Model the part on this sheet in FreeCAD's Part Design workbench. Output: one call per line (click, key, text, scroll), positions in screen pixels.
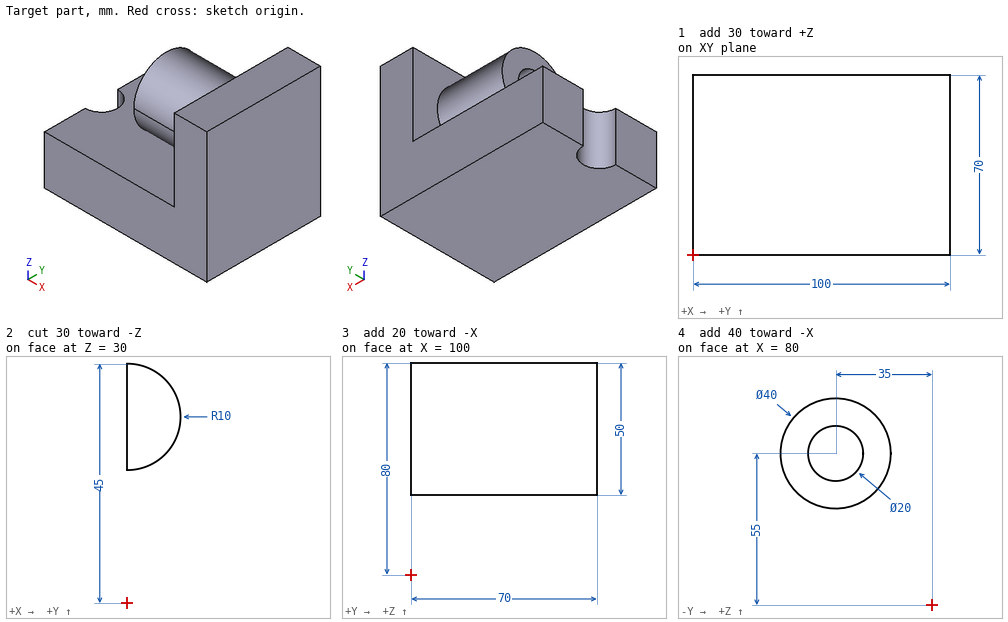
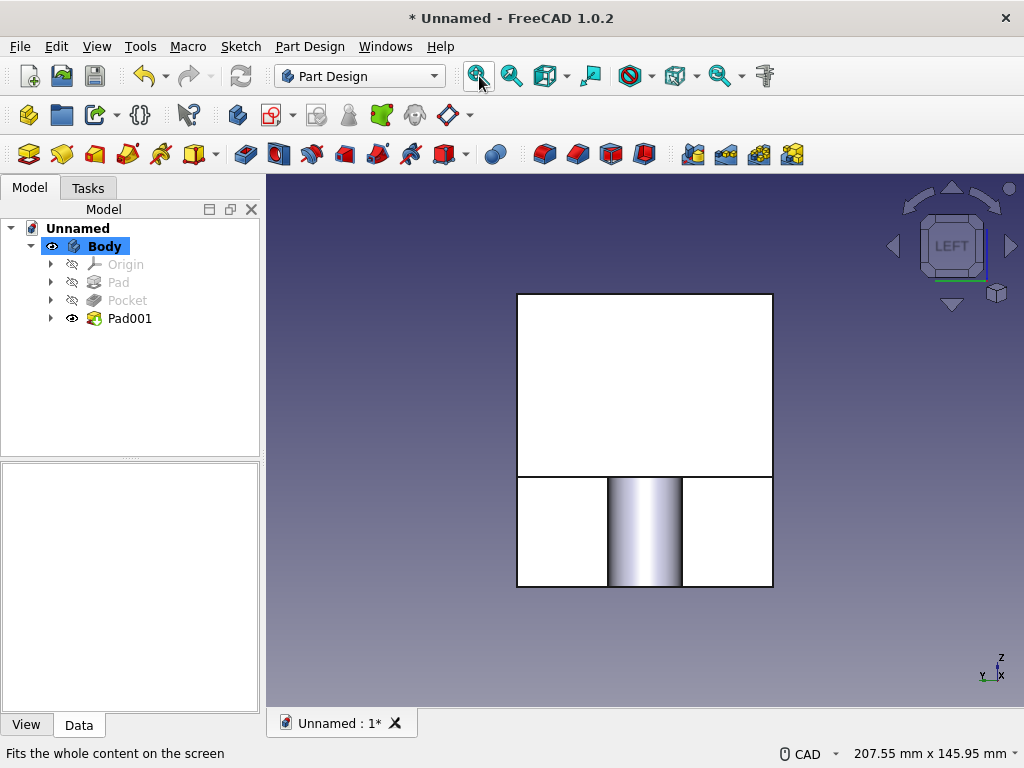
click(608, 385)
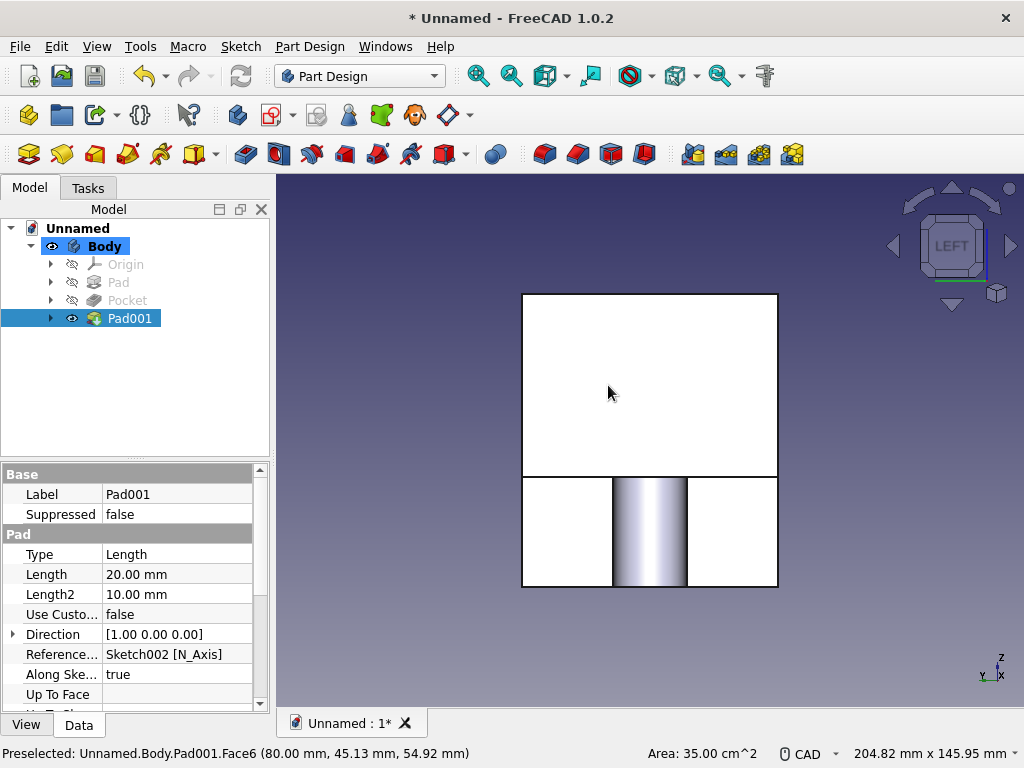
click(270, 116)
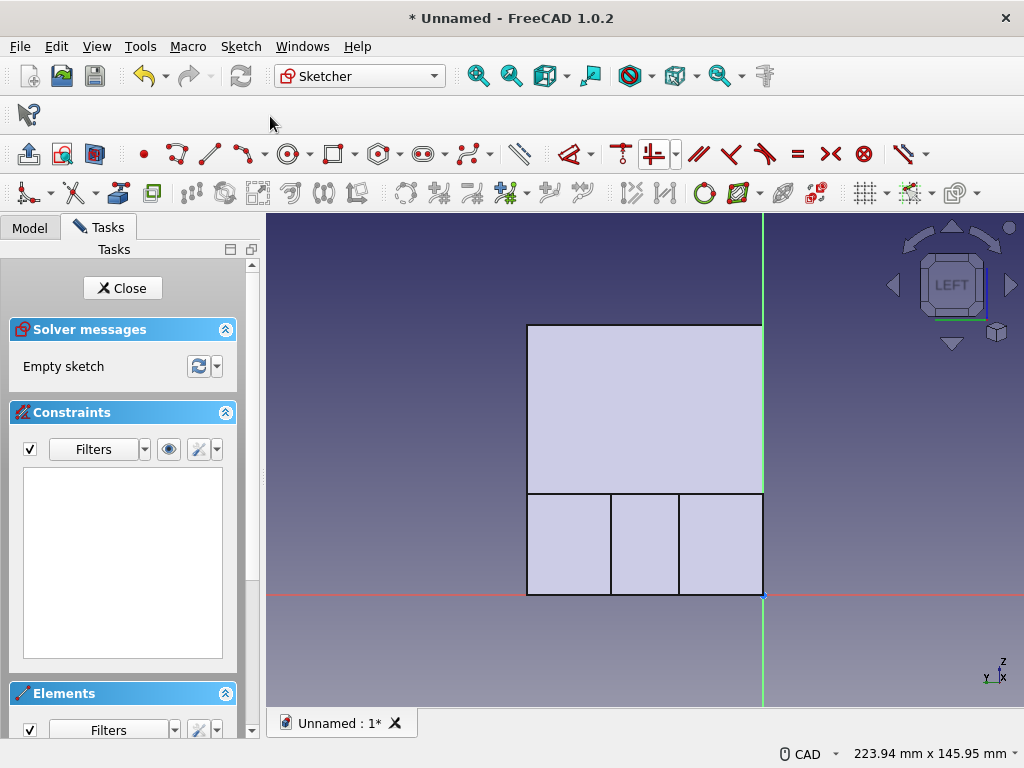
key(g)
key(c)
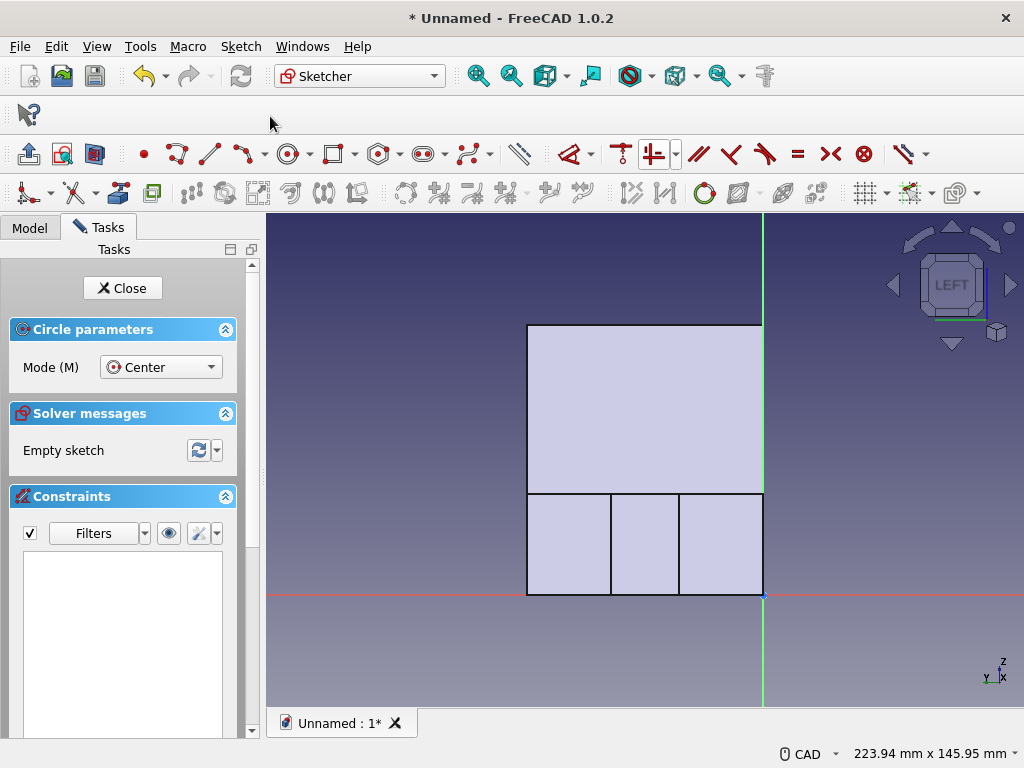
click(645, 409)
move(693, 361)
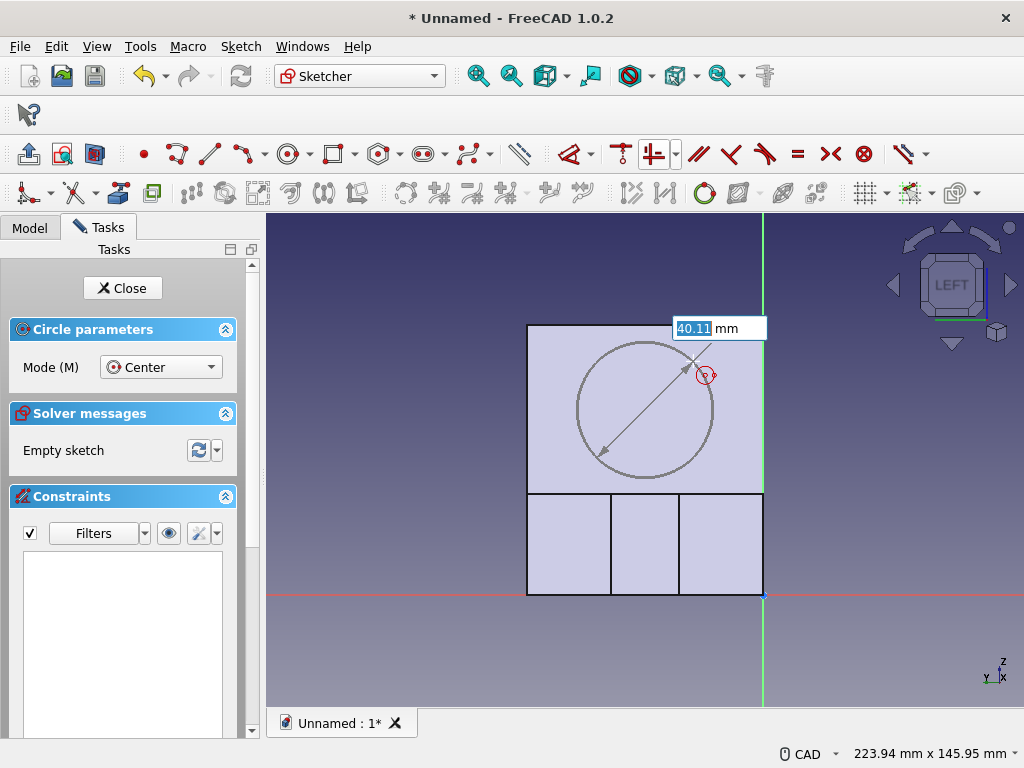
text(40)
key(Return)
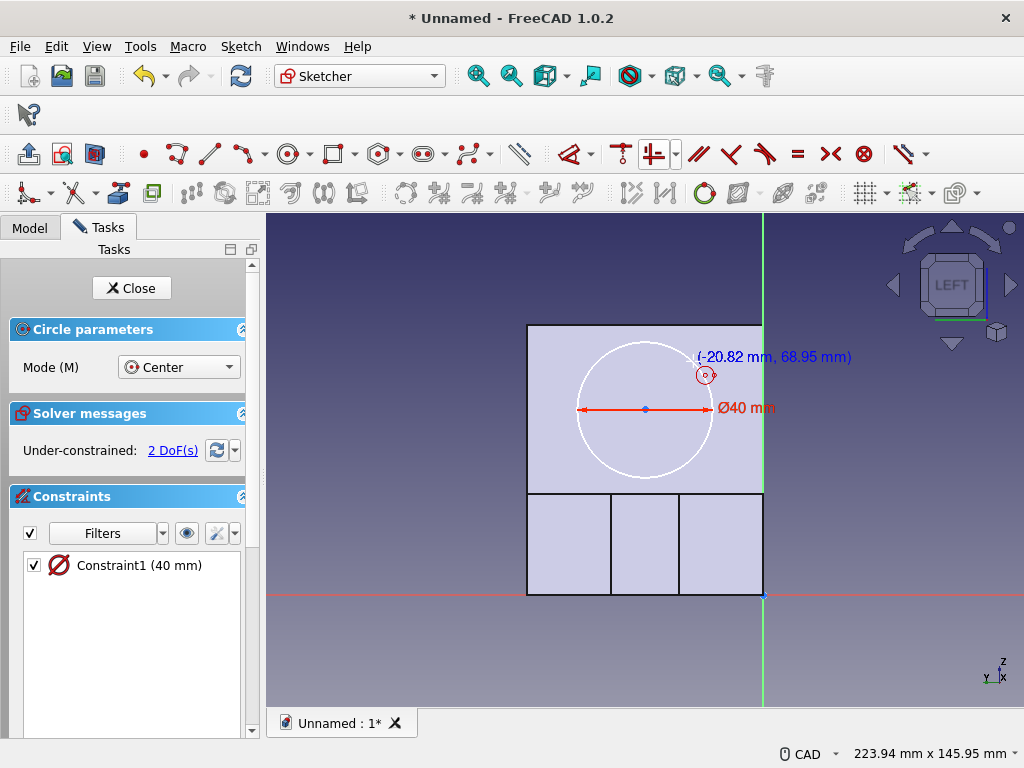
click(645, 410)
move(669, 385)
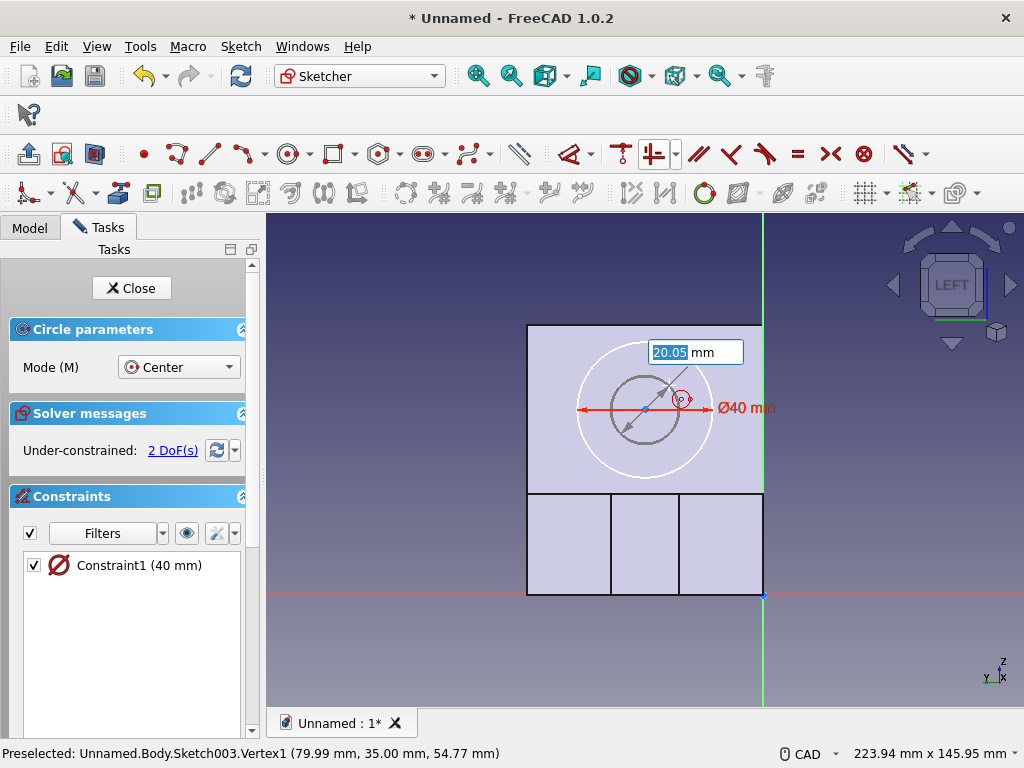
text(20)
key(Return)
key(Escape)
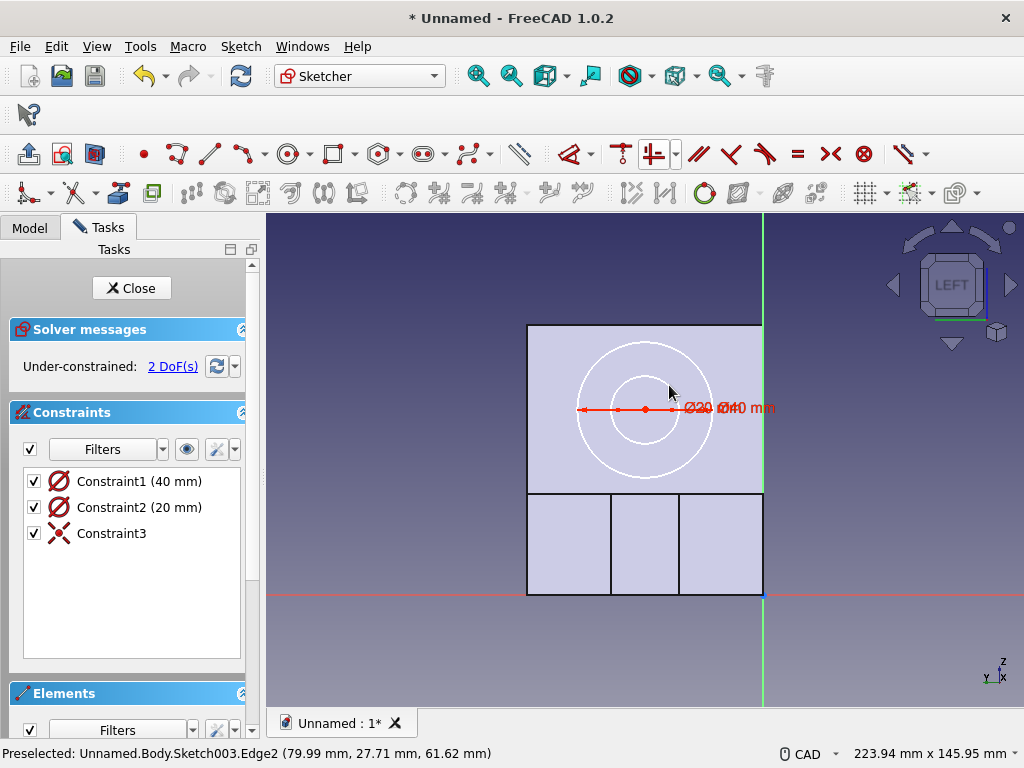
click(568, 154)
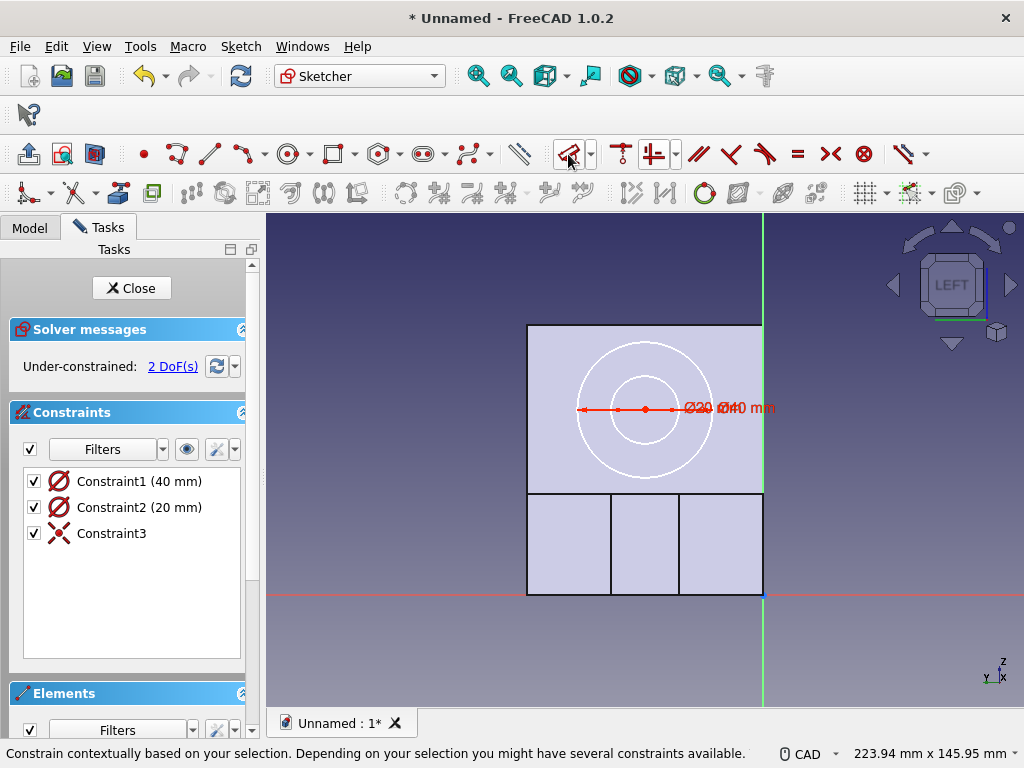
click(645, 410)
click(704, 629)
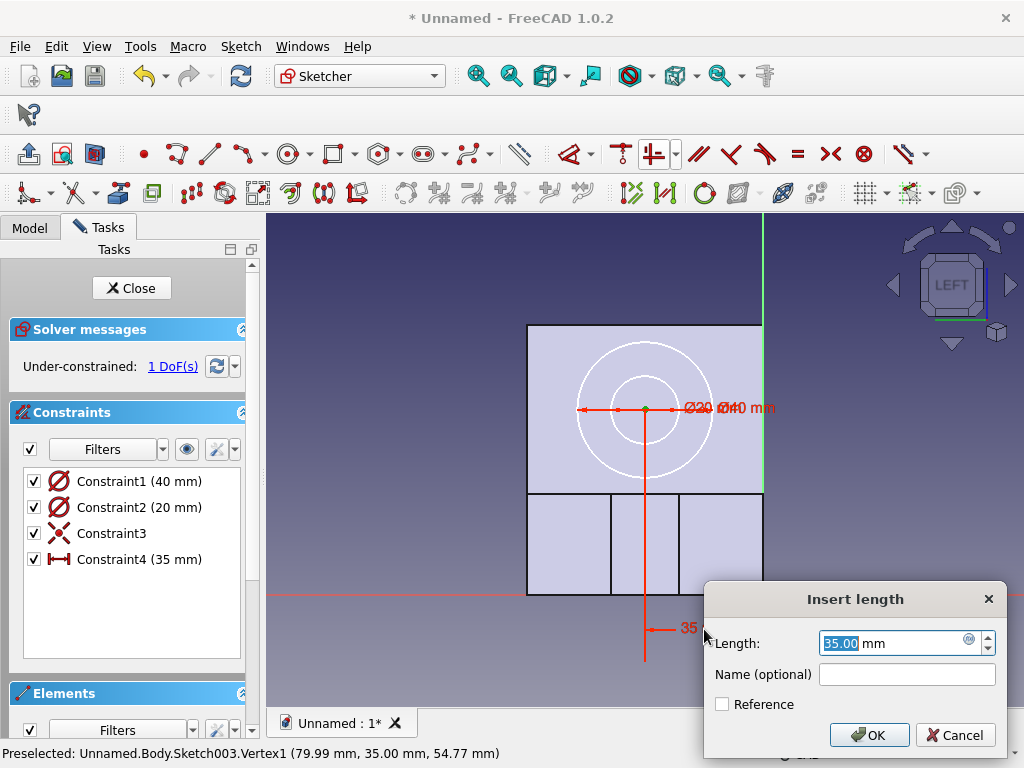
text(35)
key(Return)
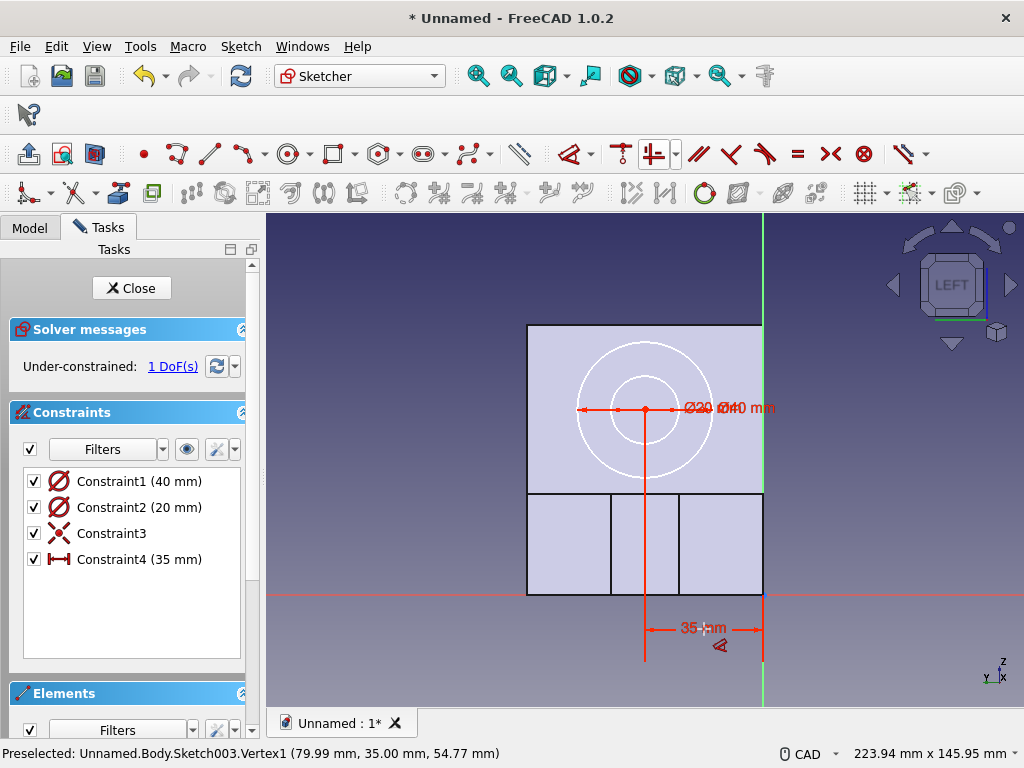
click(645, 410)
click(797, 503)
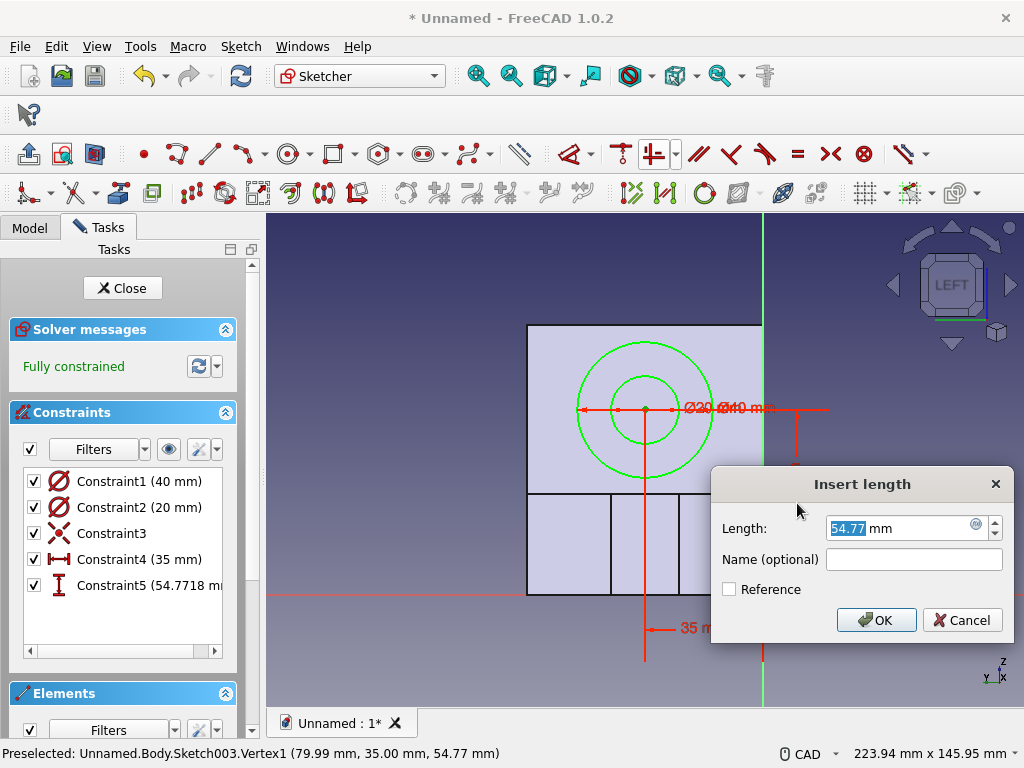
text(55)
key(Return)
key(Escape)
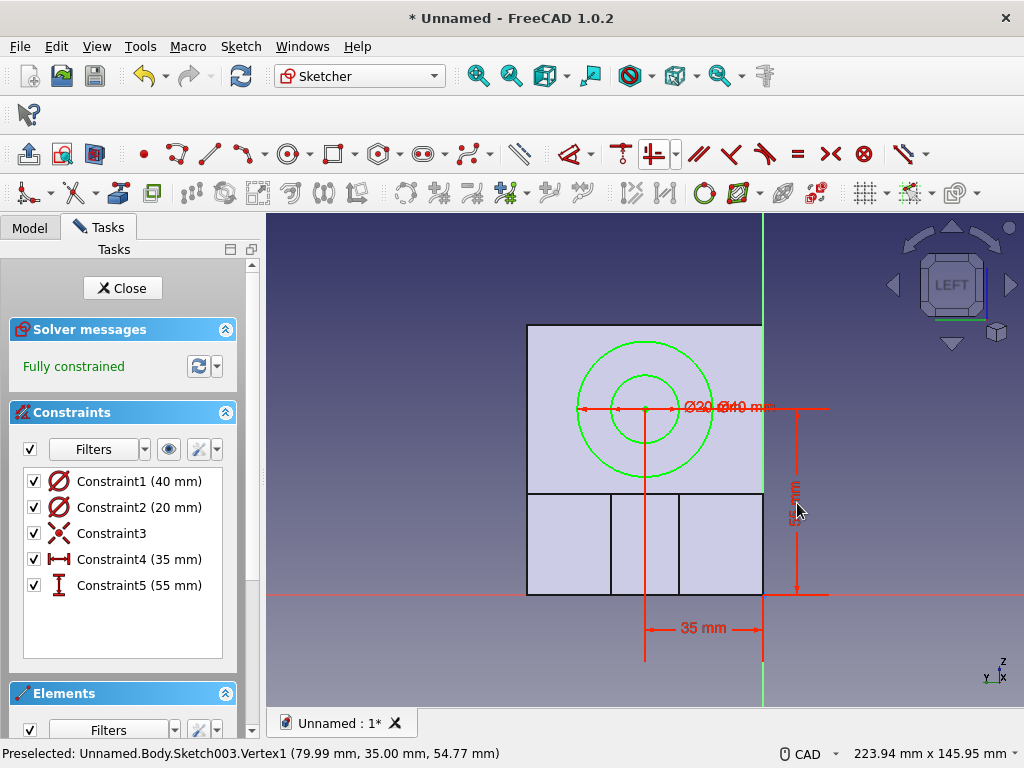
click(123, 288)